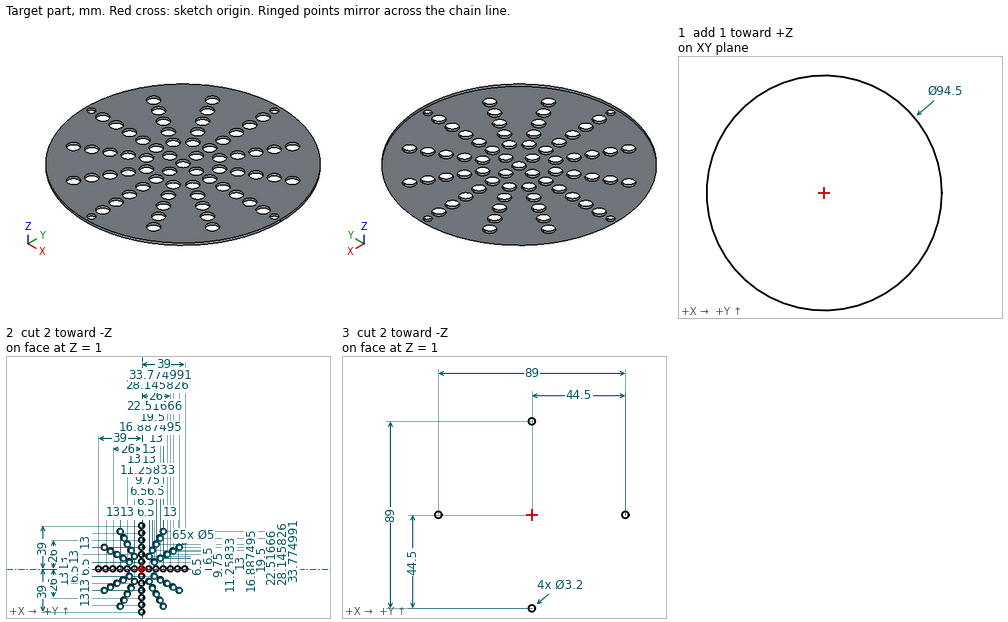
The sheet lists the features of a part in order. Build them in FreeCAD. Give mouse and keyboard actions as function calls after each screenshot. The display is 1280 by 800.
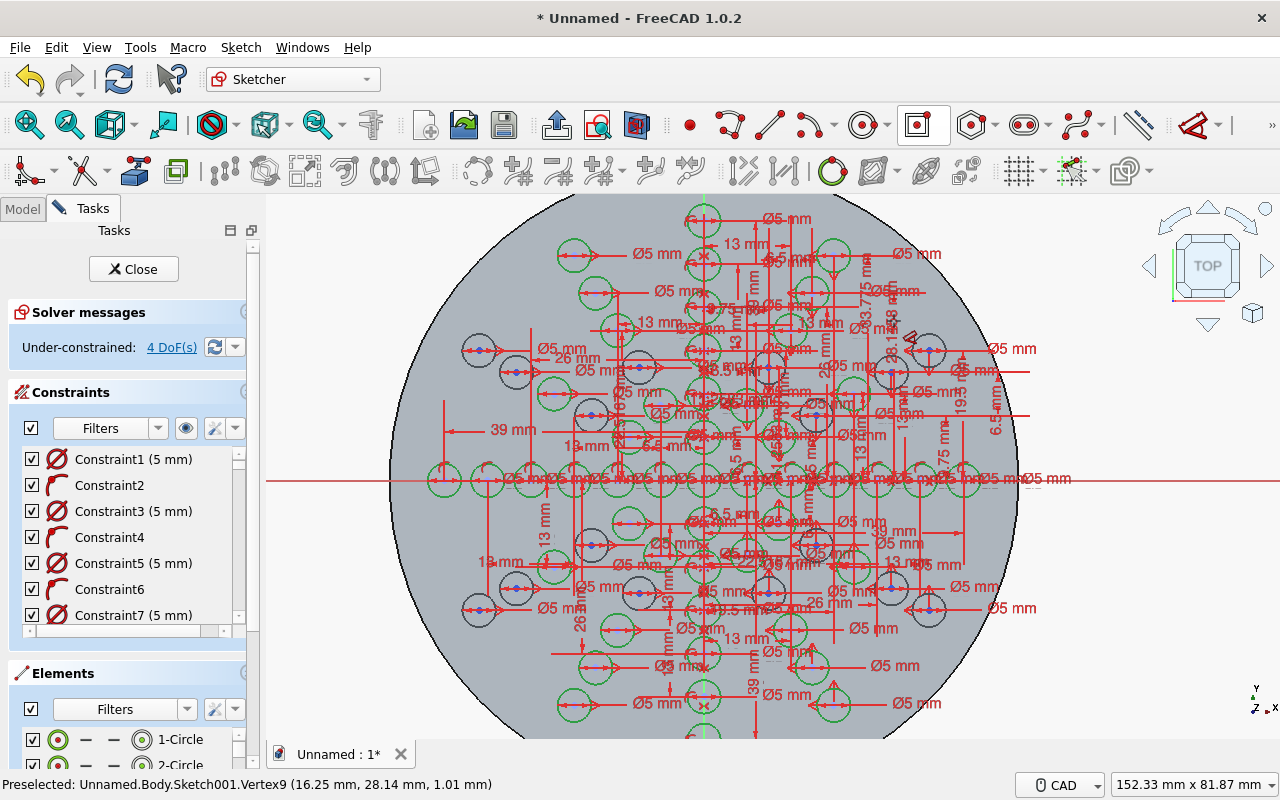
click(769, 368)
click(598, 385)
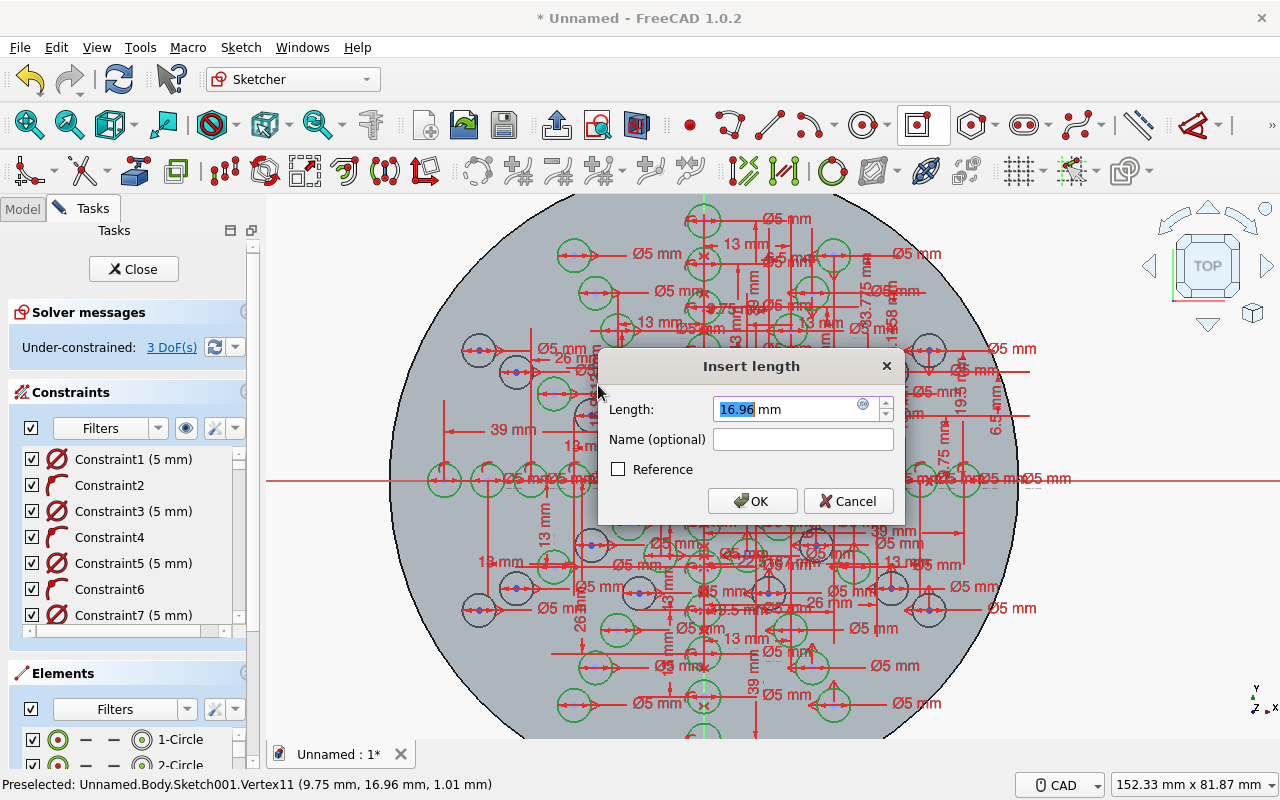
text(16.887495)
key(Return)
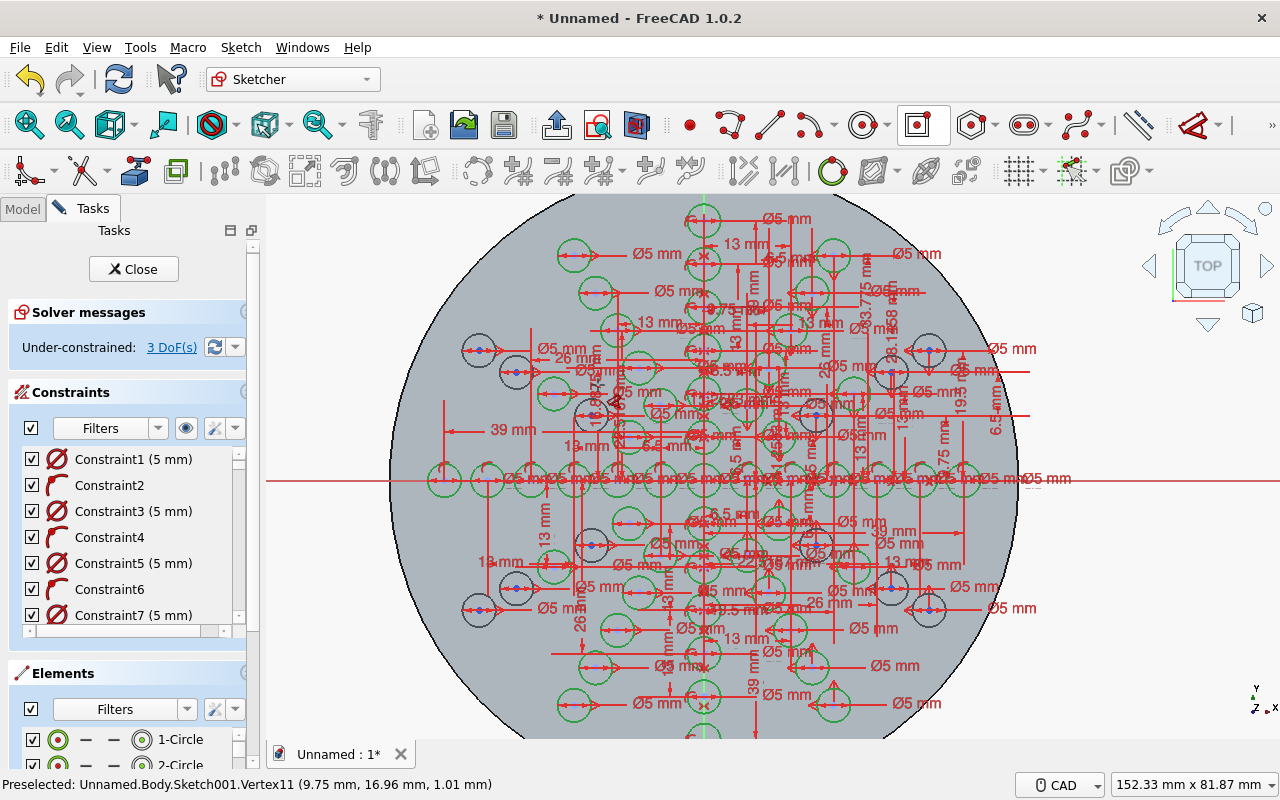
click(929, 351)
click(868, 269)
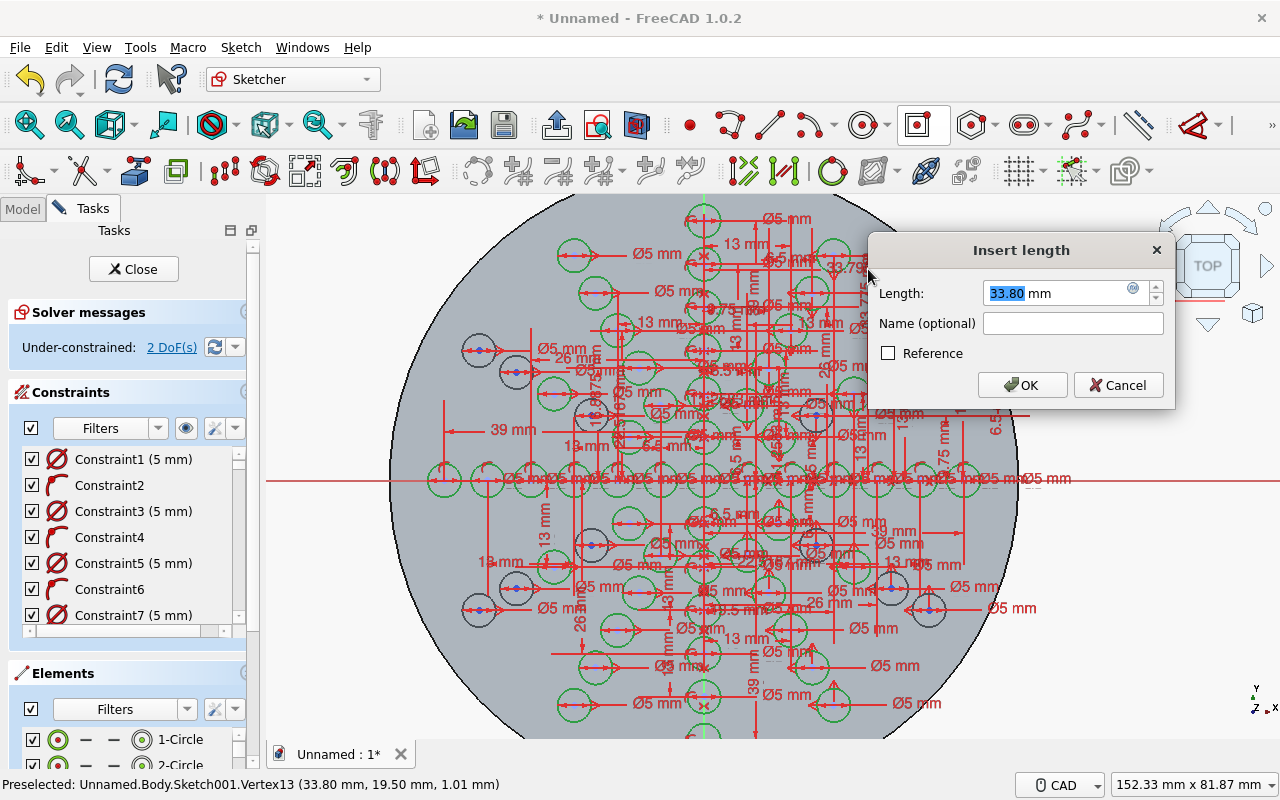
text(33.774991)
key(Return)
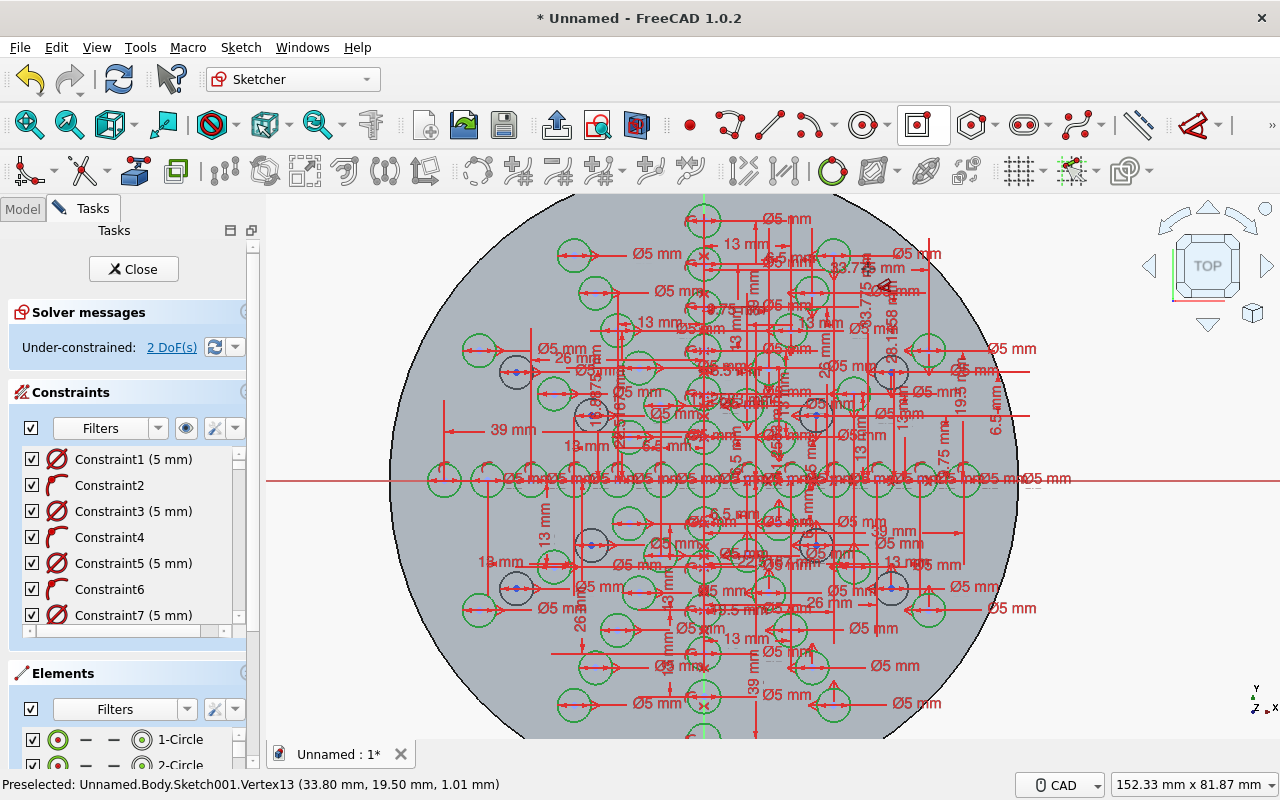
click(892, 372)
click(863, 242)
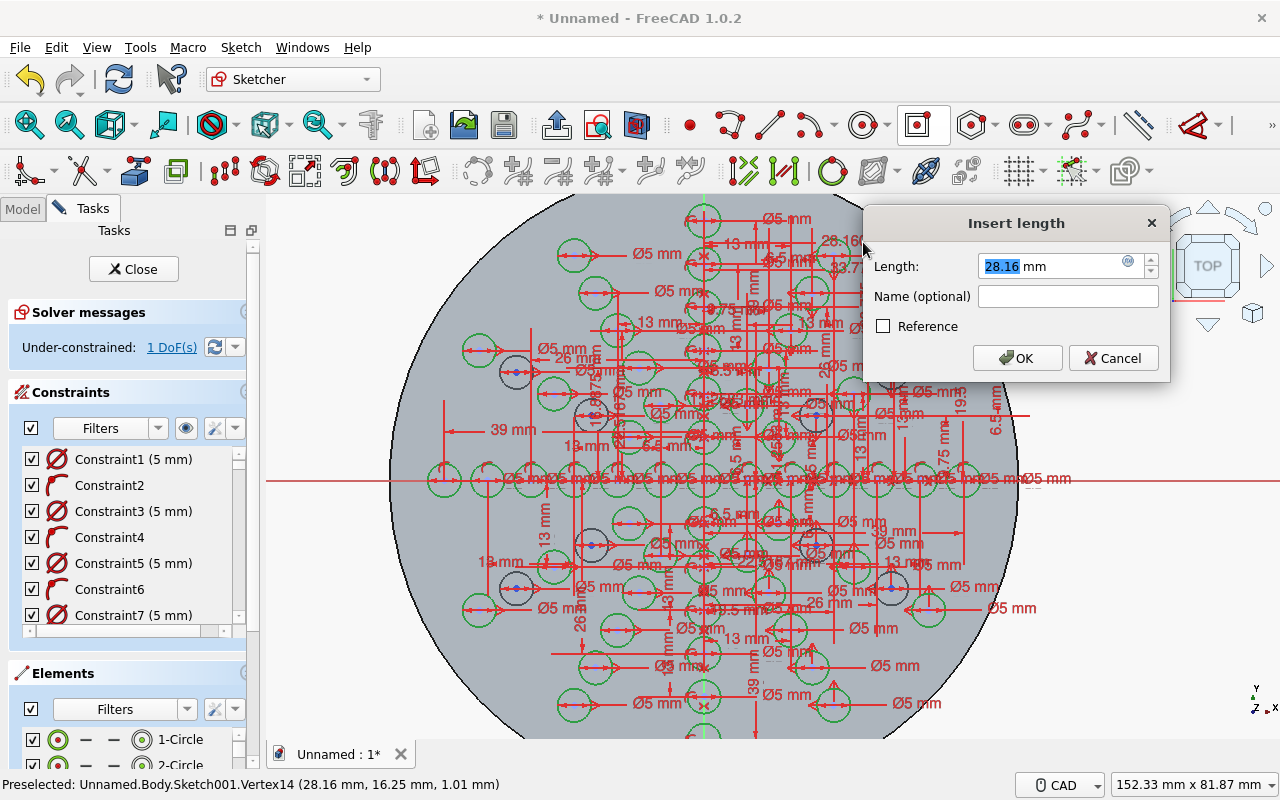
text(28.145826)
key(Return)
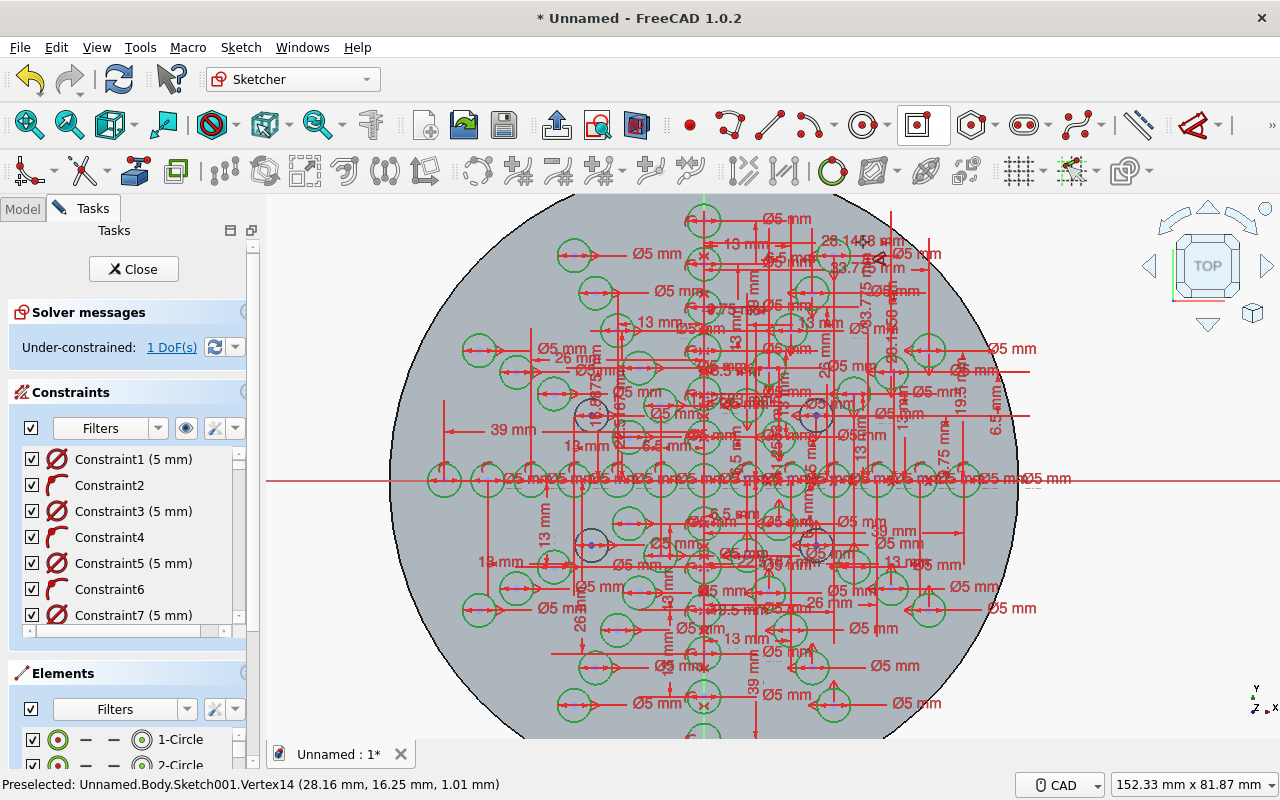
click(816, 416)
click(800, 382)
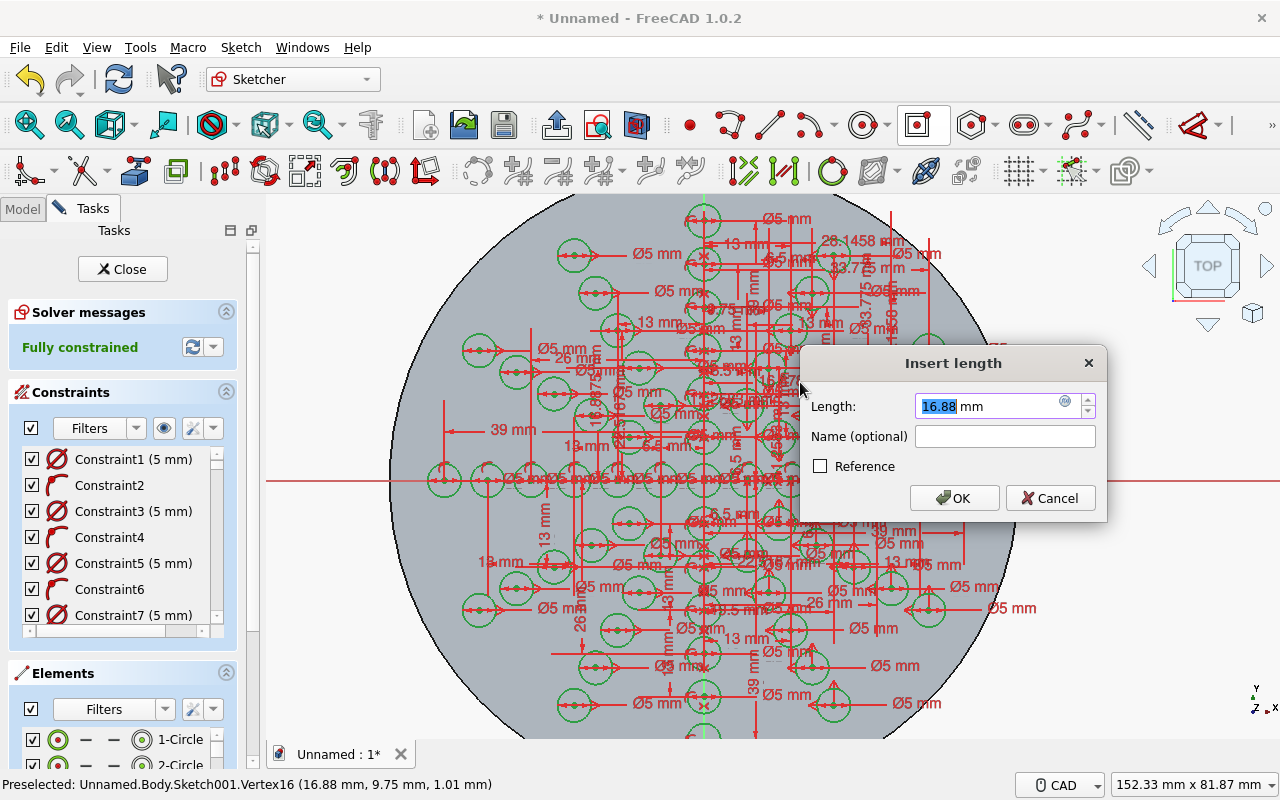
text(16.887495)
key(Return)
key(Escape)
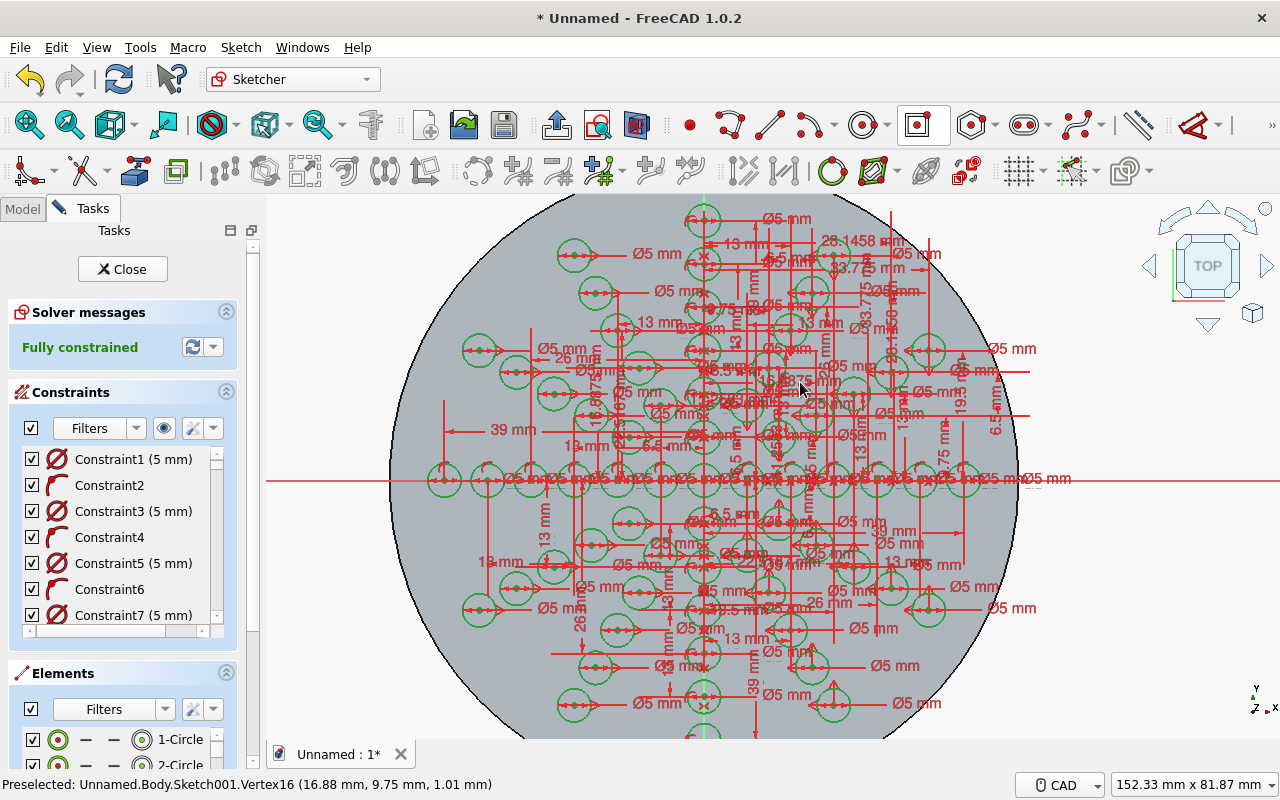
click(123, 269)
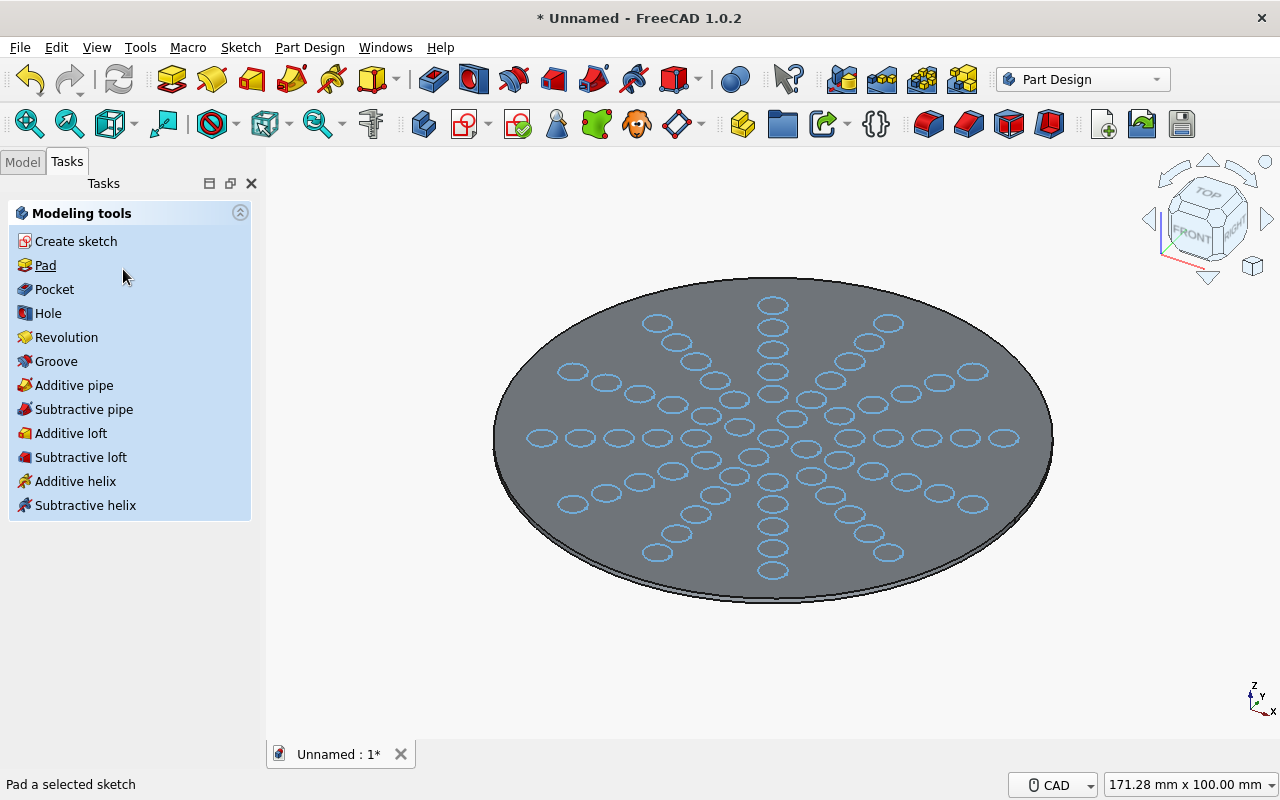
click(434, 80)